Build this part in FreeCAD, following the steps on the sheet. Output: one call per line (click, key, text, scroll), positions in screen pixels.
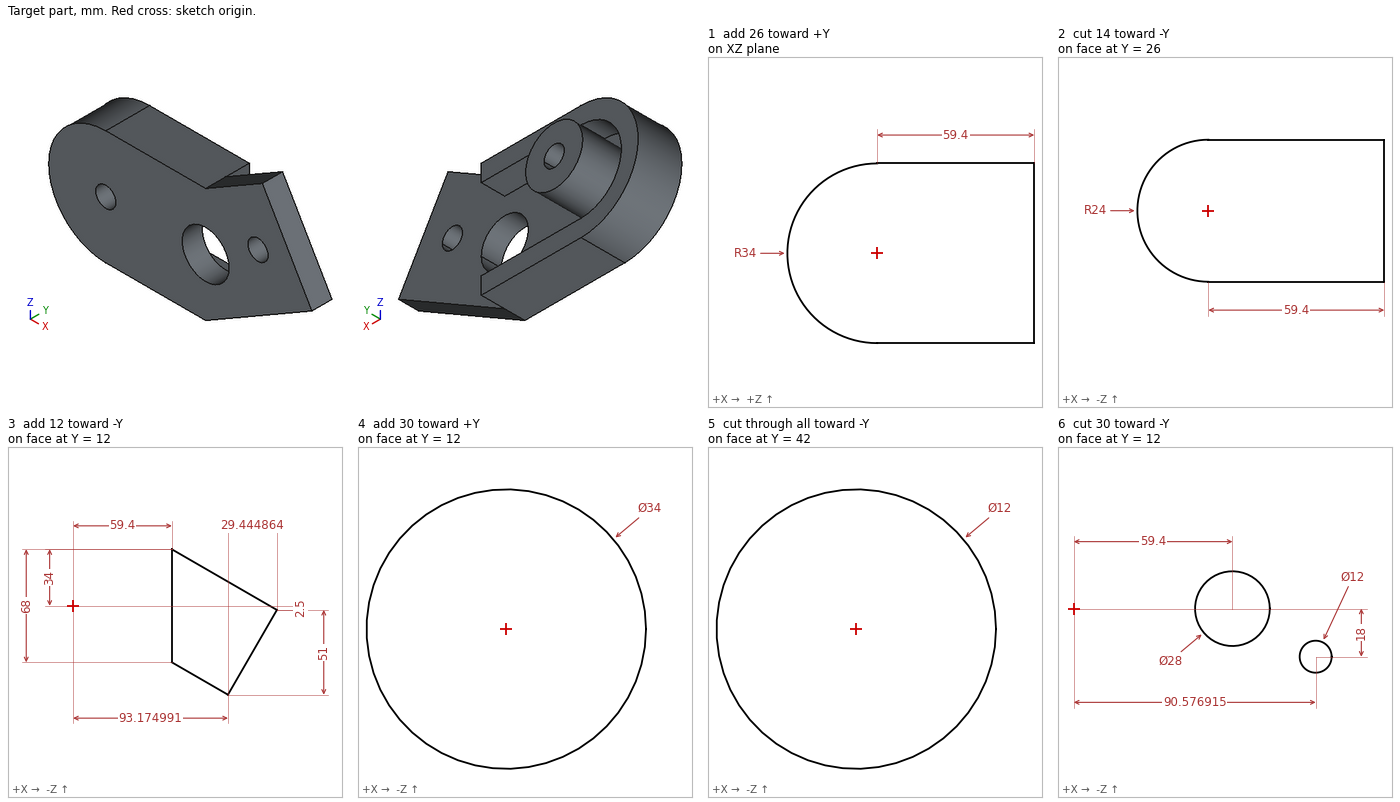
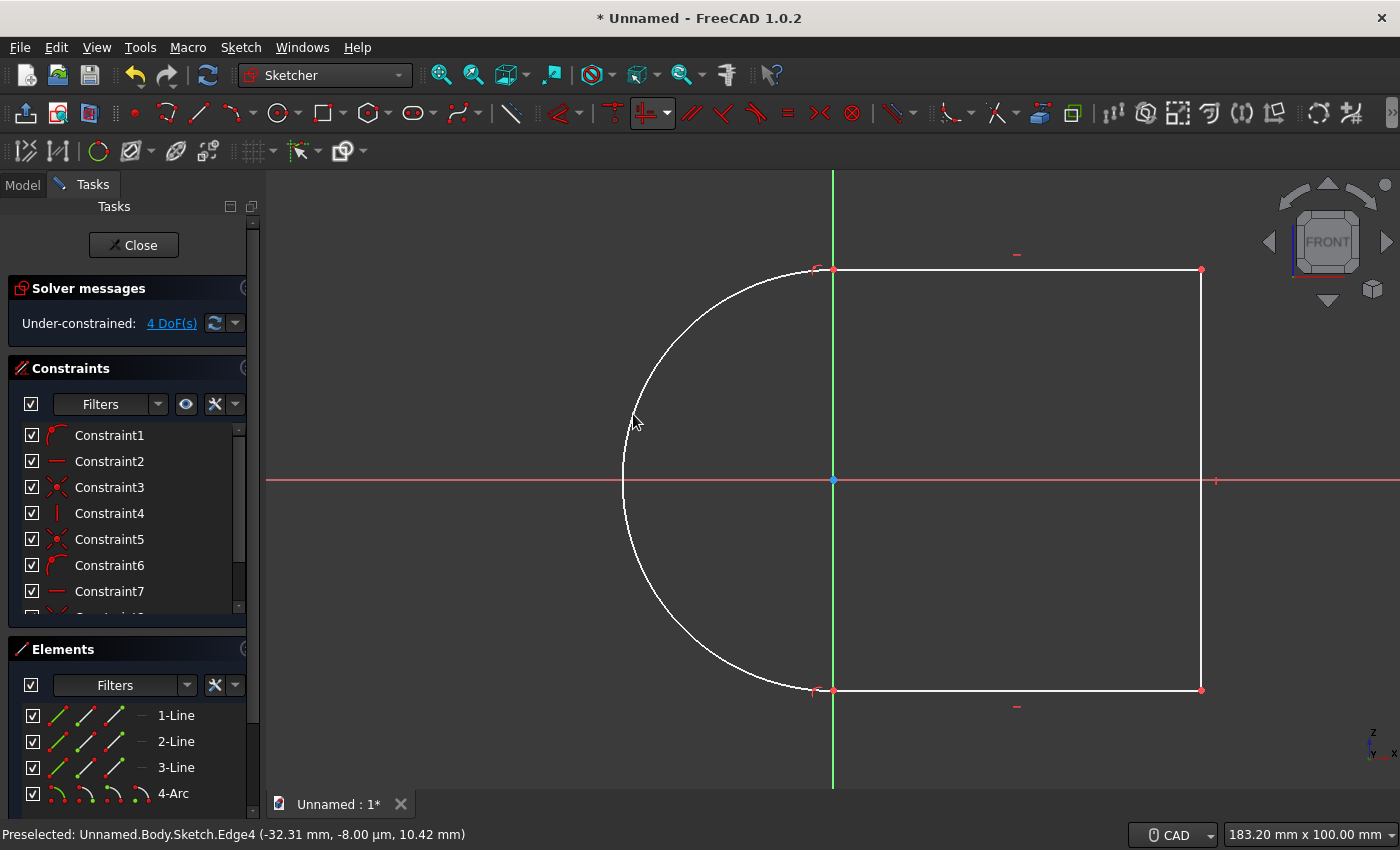
drag(823, 470, 843, 490)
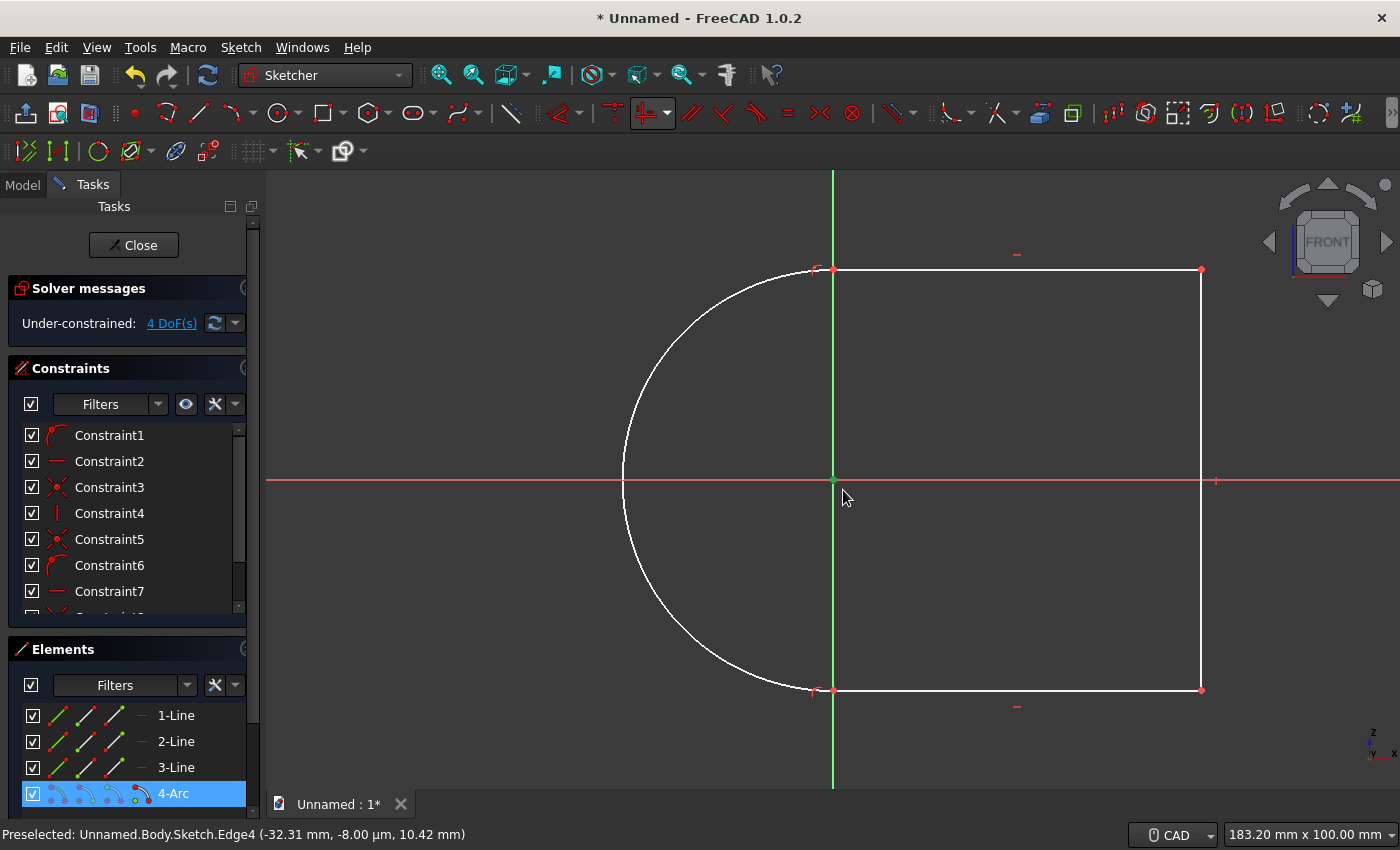
click(614, 114)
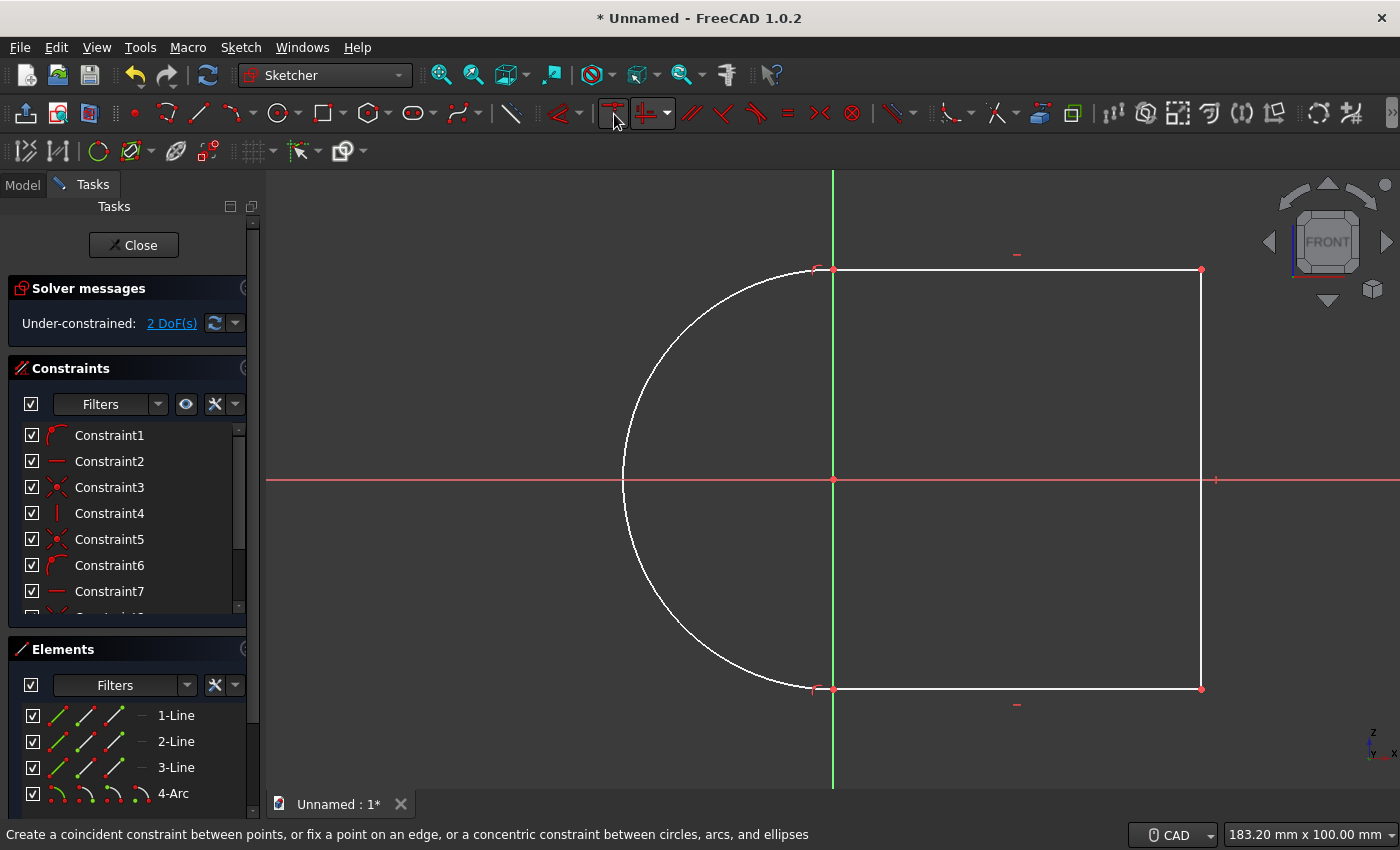
click(663, 356)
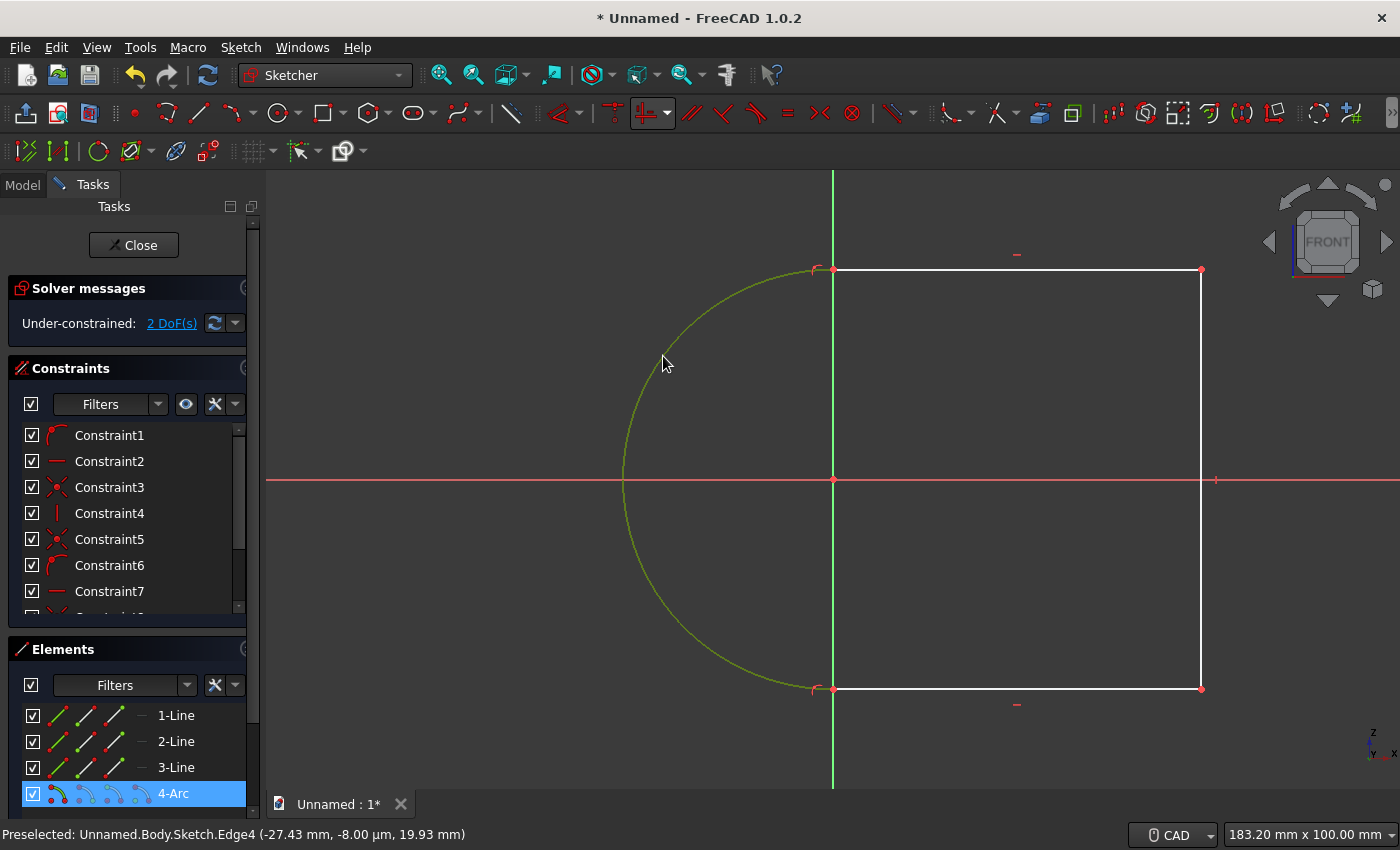
click(582, 114)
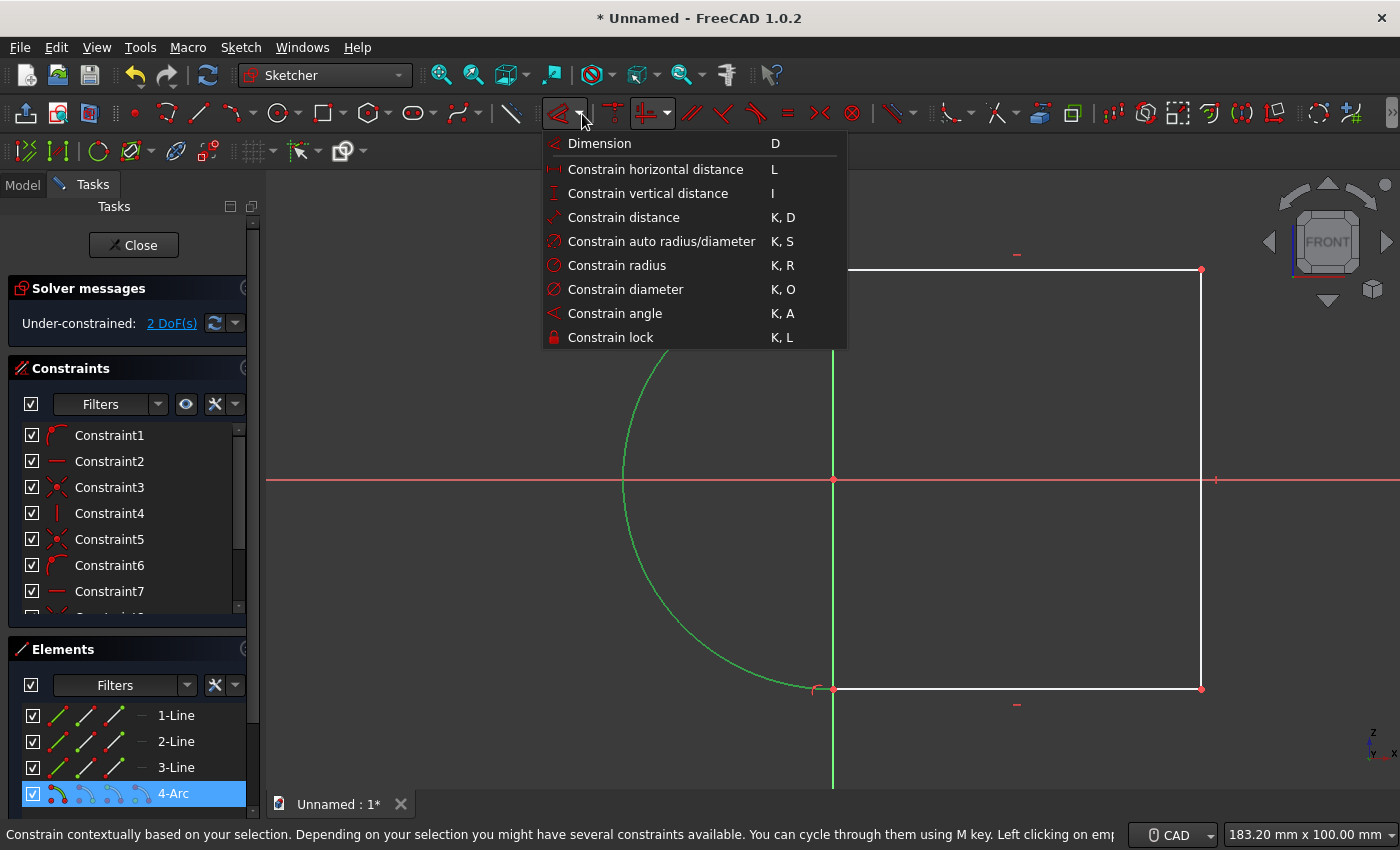
click(695, 265)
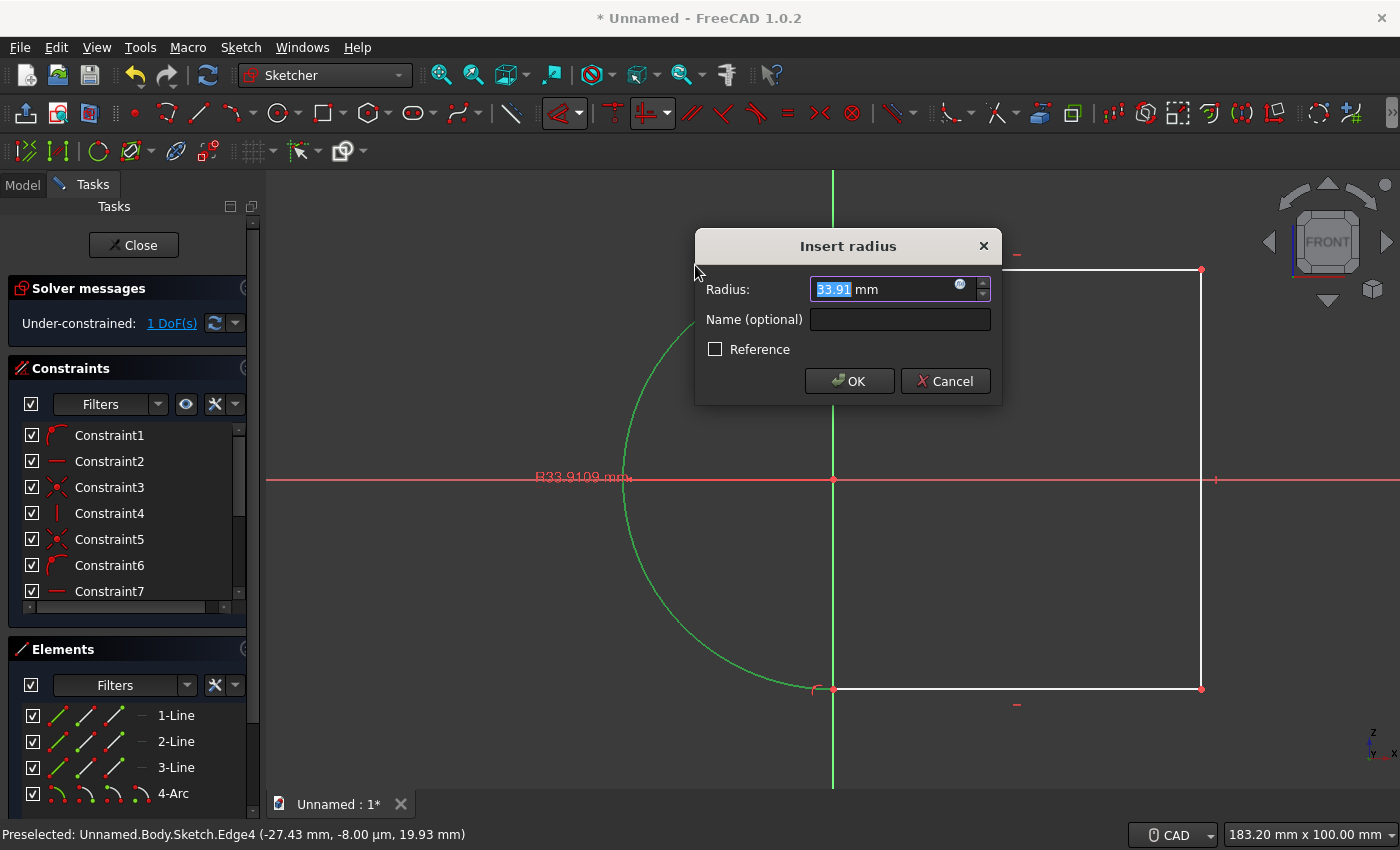
text(34)
key(Return)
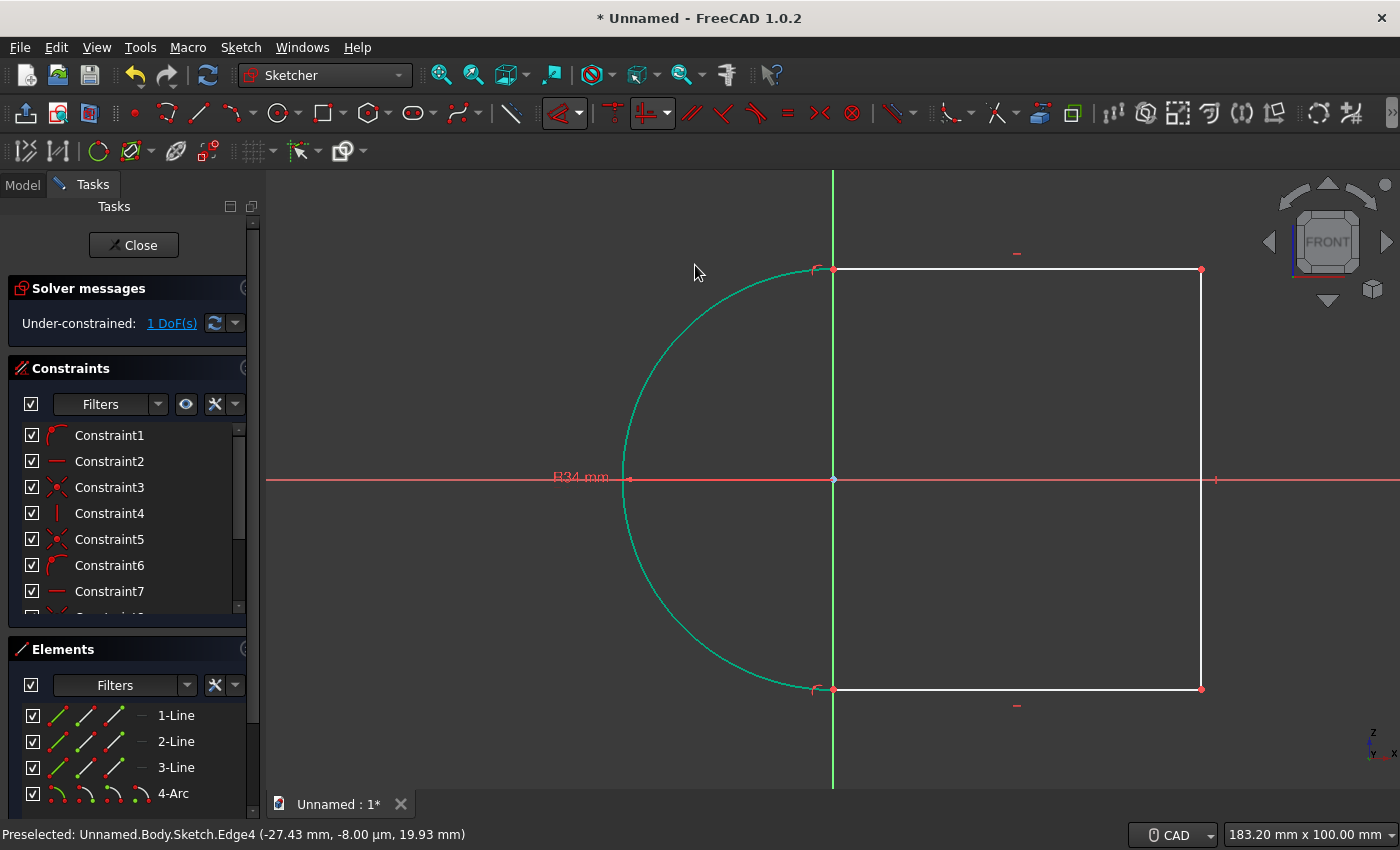
click(943, 269)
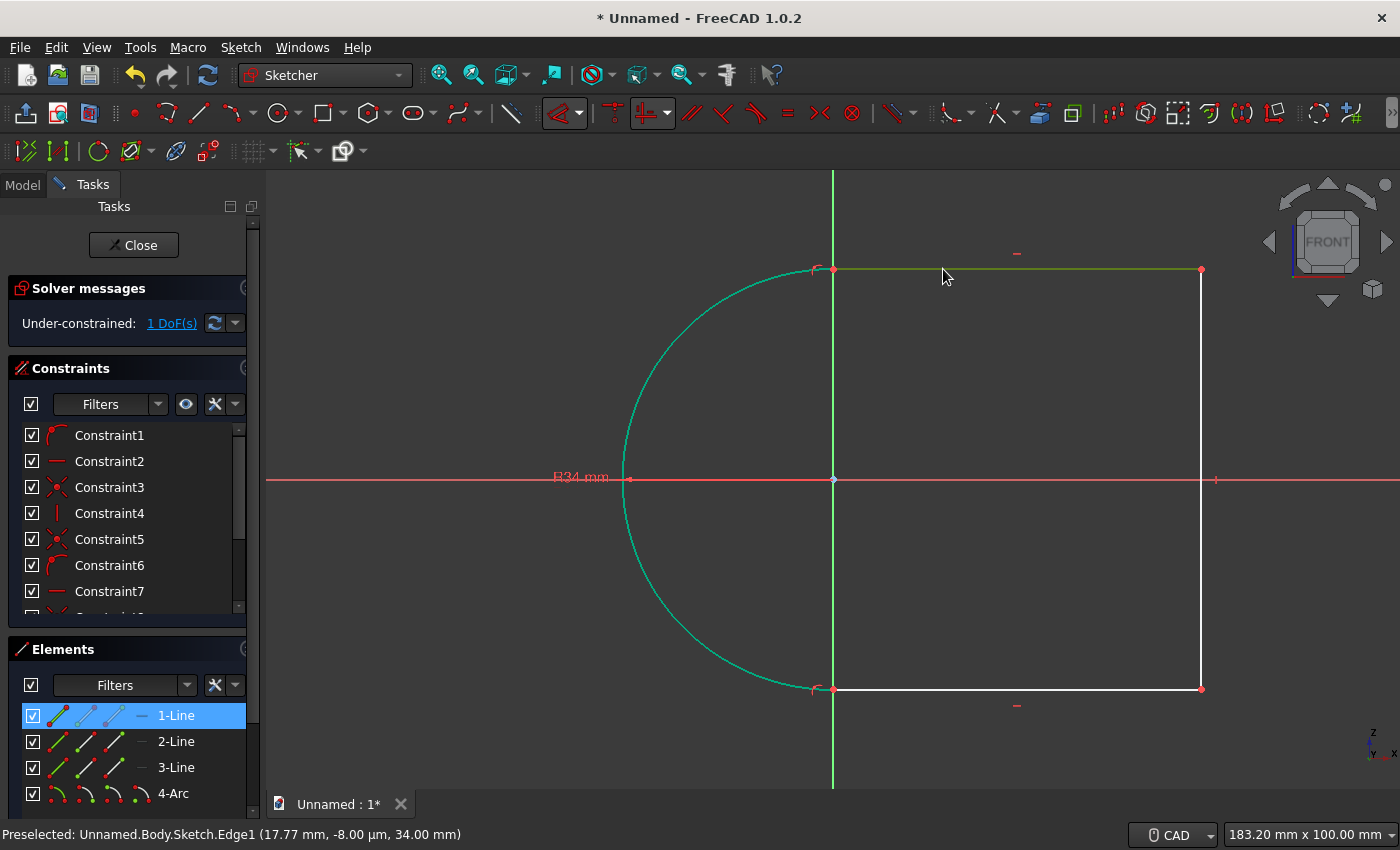
key(l)